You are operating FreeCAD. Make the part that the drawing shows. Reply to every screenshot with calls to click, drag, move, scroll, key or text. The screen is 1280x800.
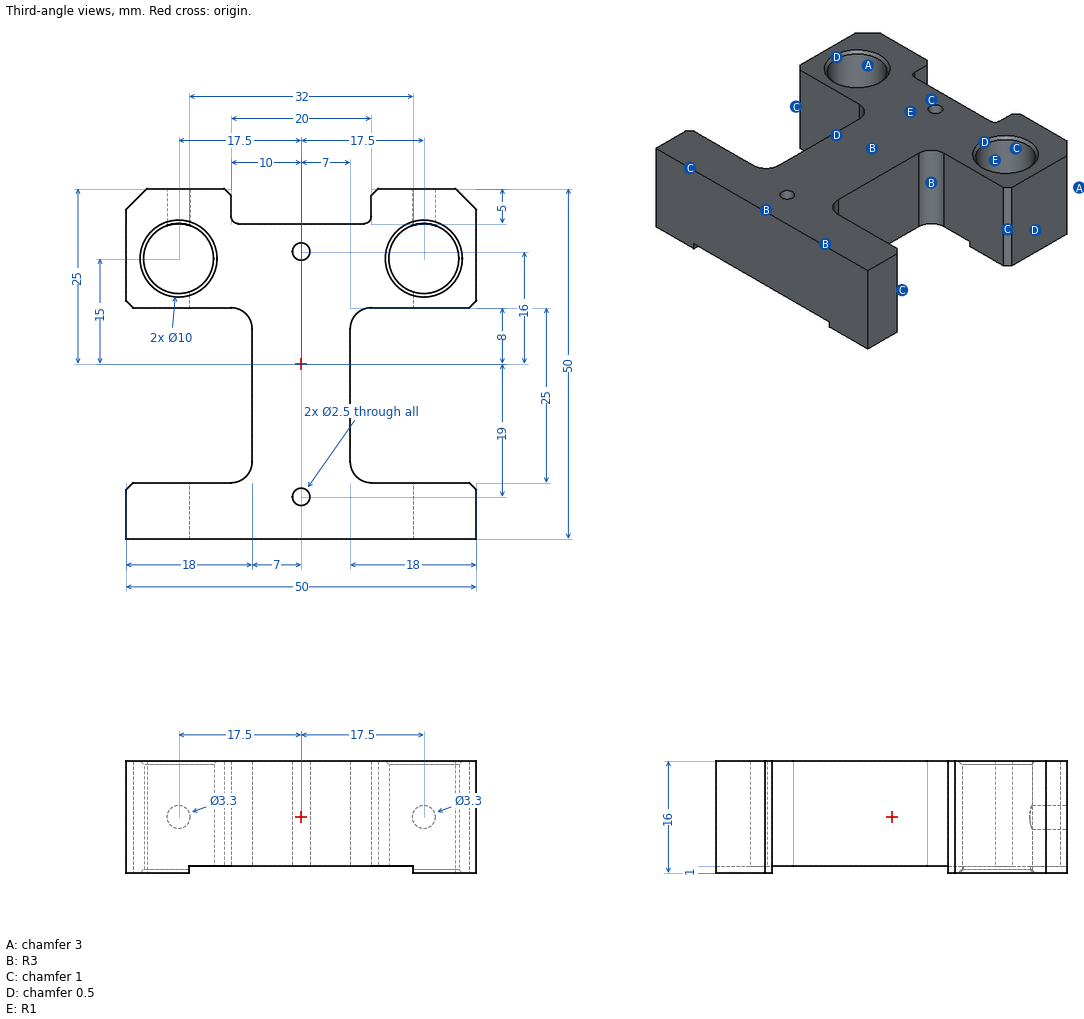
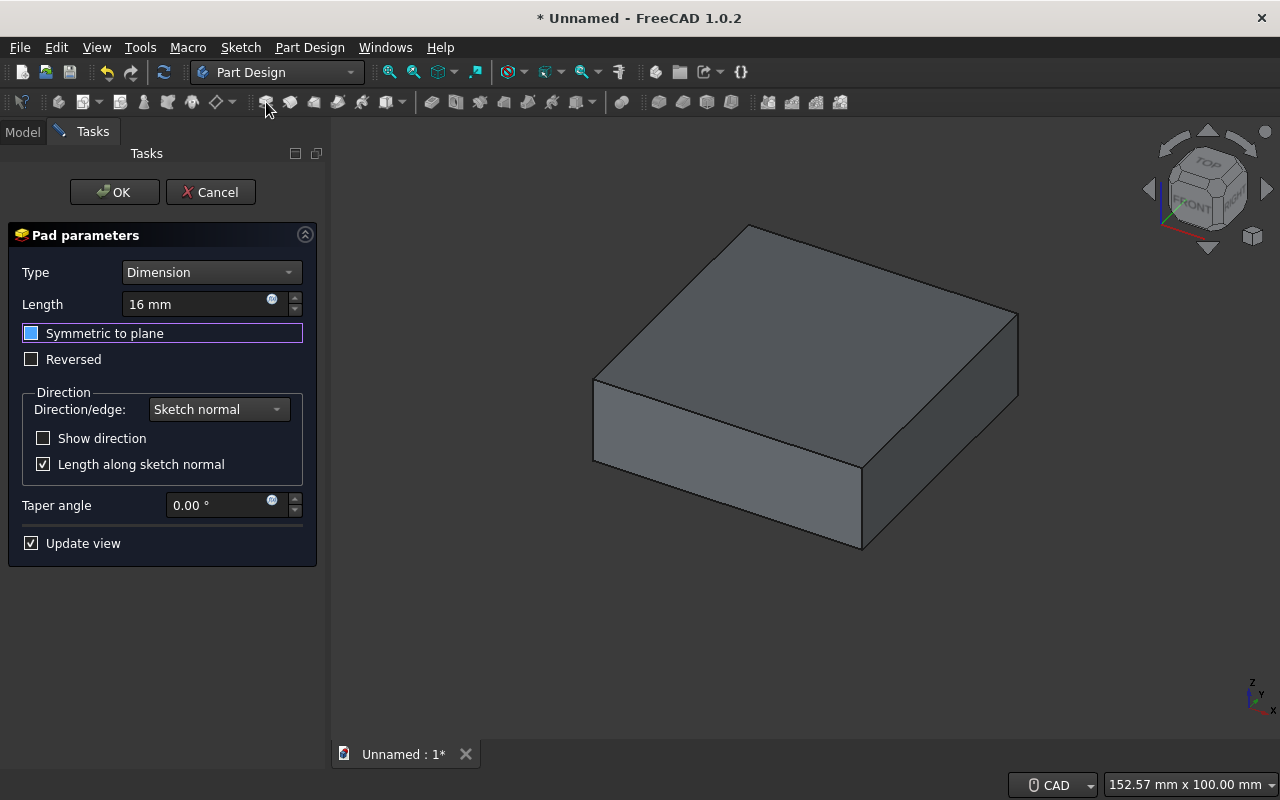
click(30, 333)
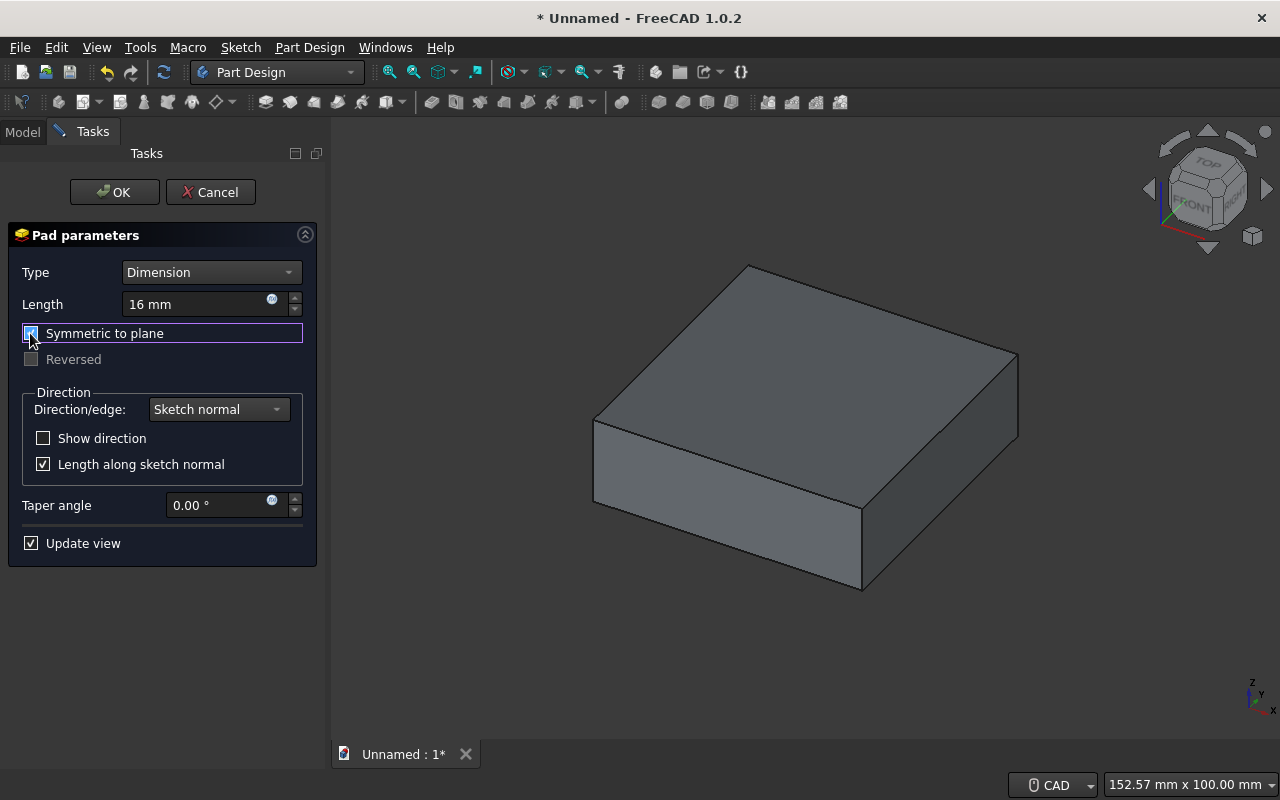
click(115, 192)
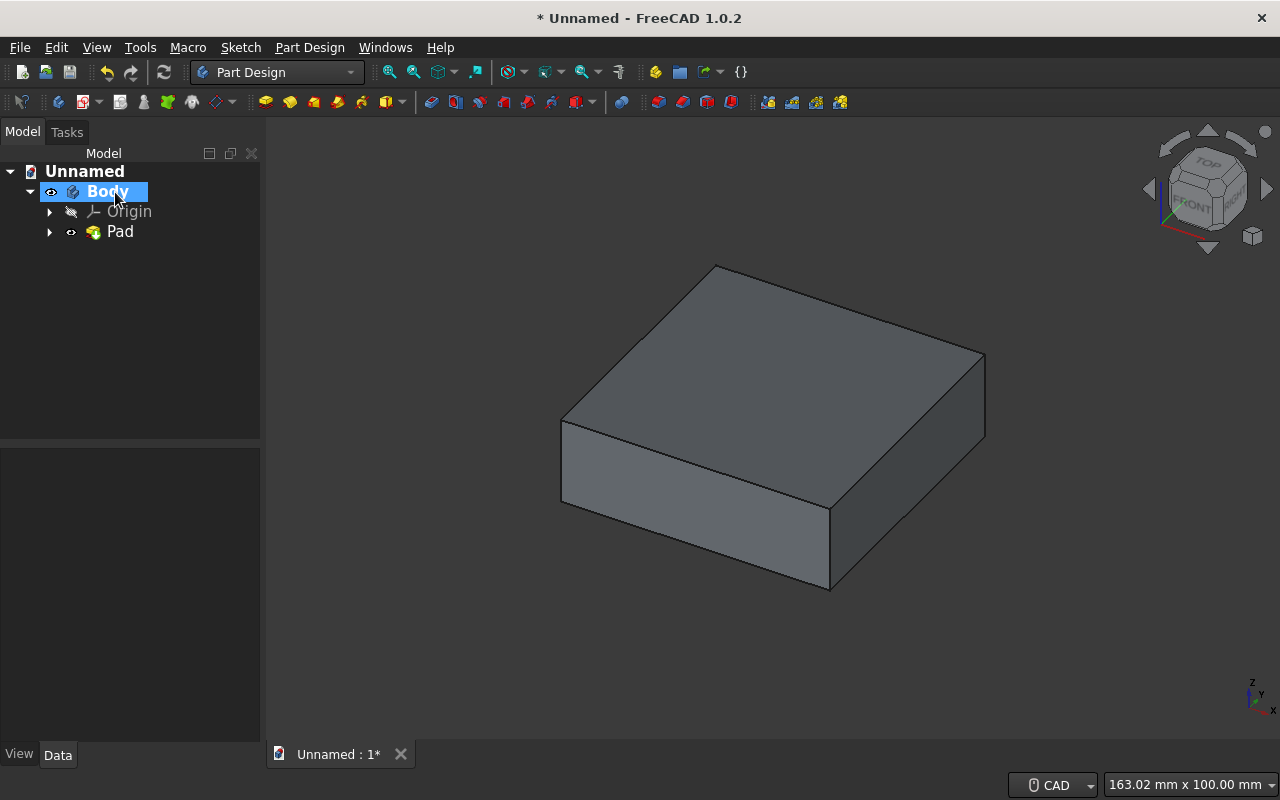
click(773, 386)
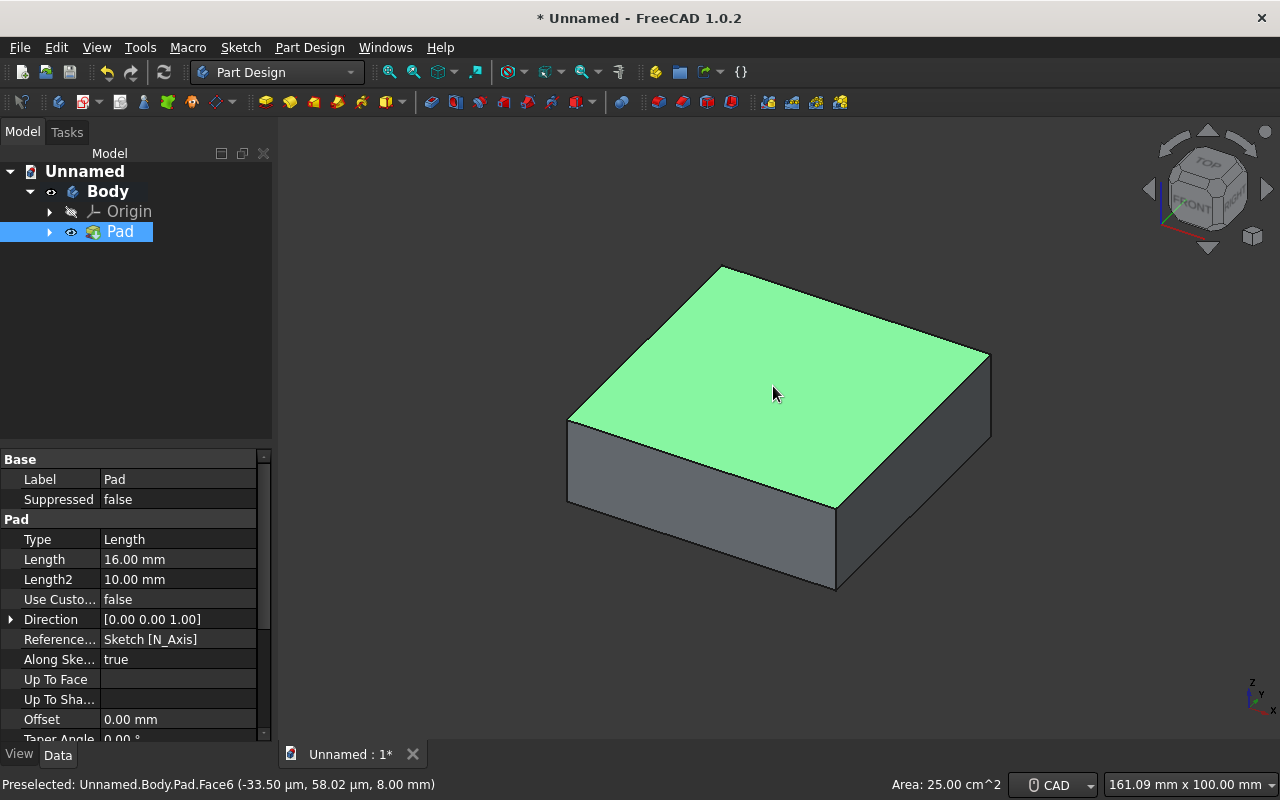
click(84, 102)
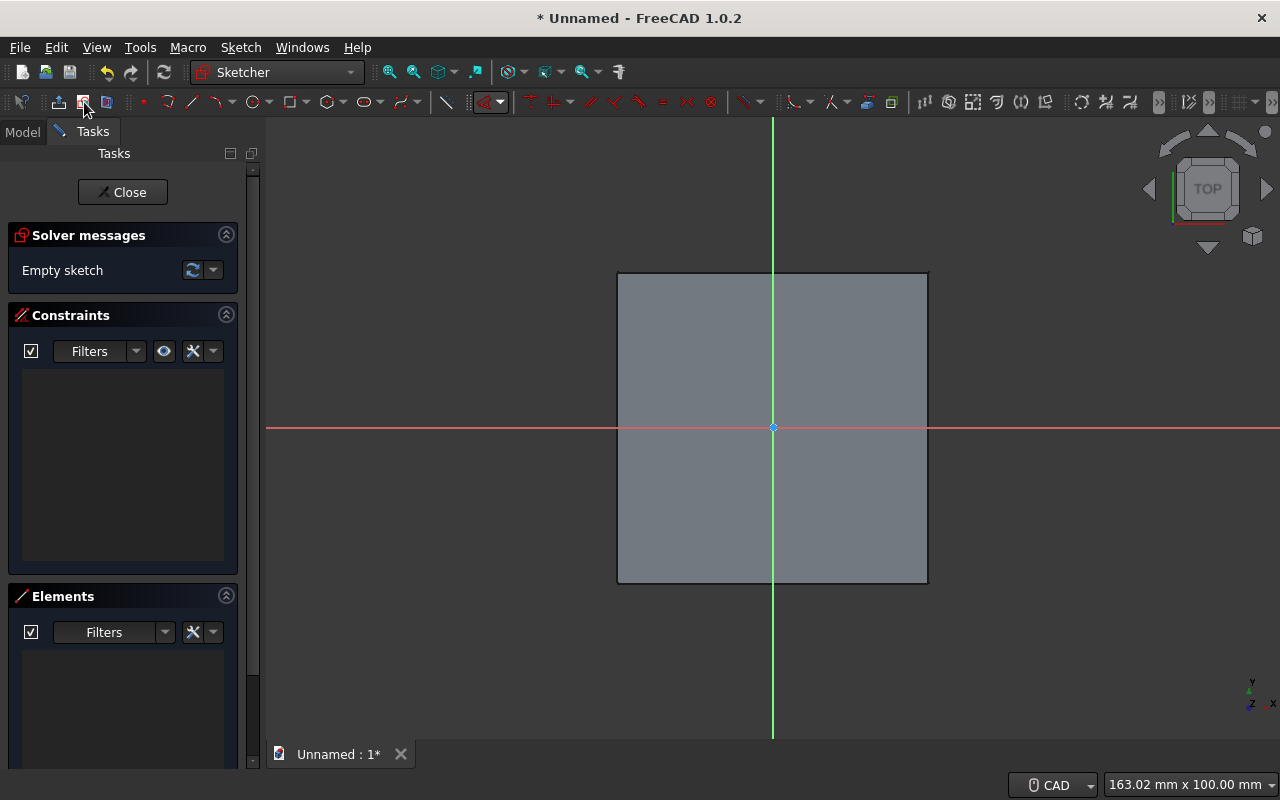
scroll(856, 407, up, 3)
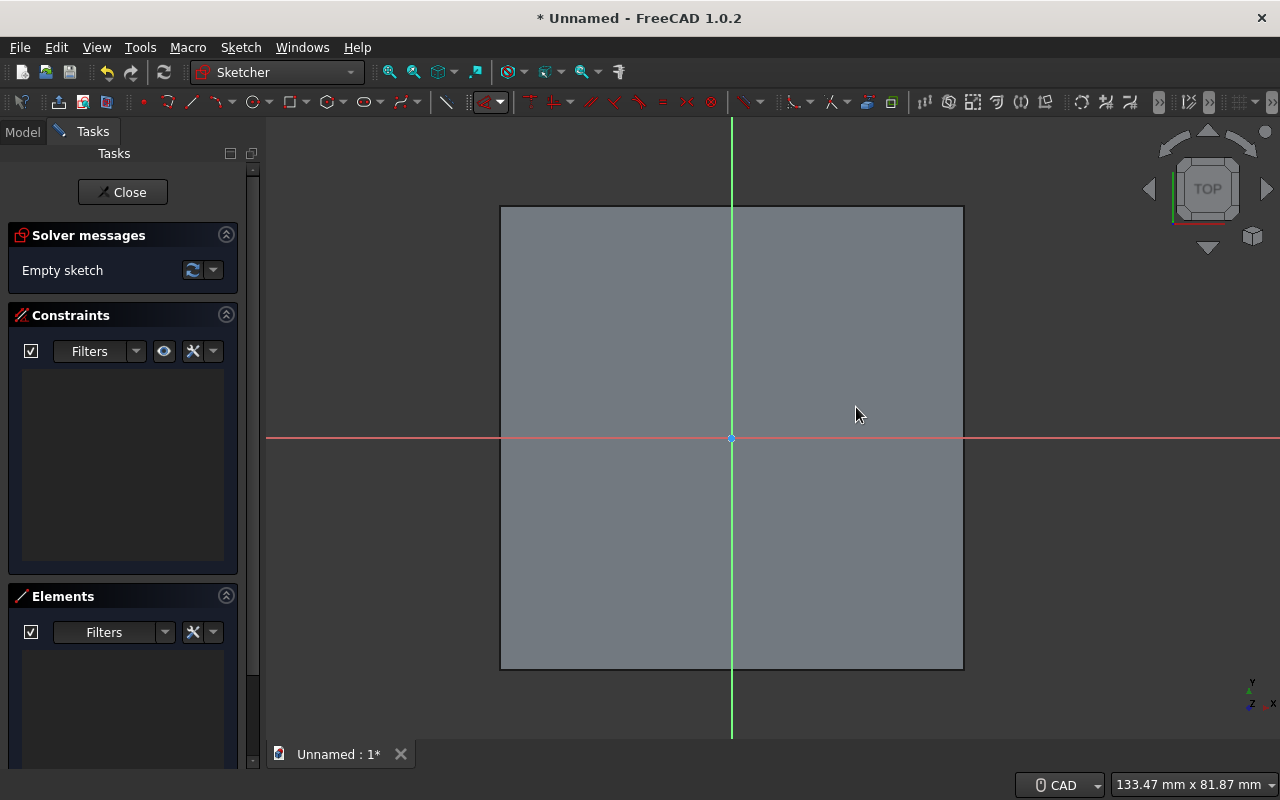
key(g)
key(r)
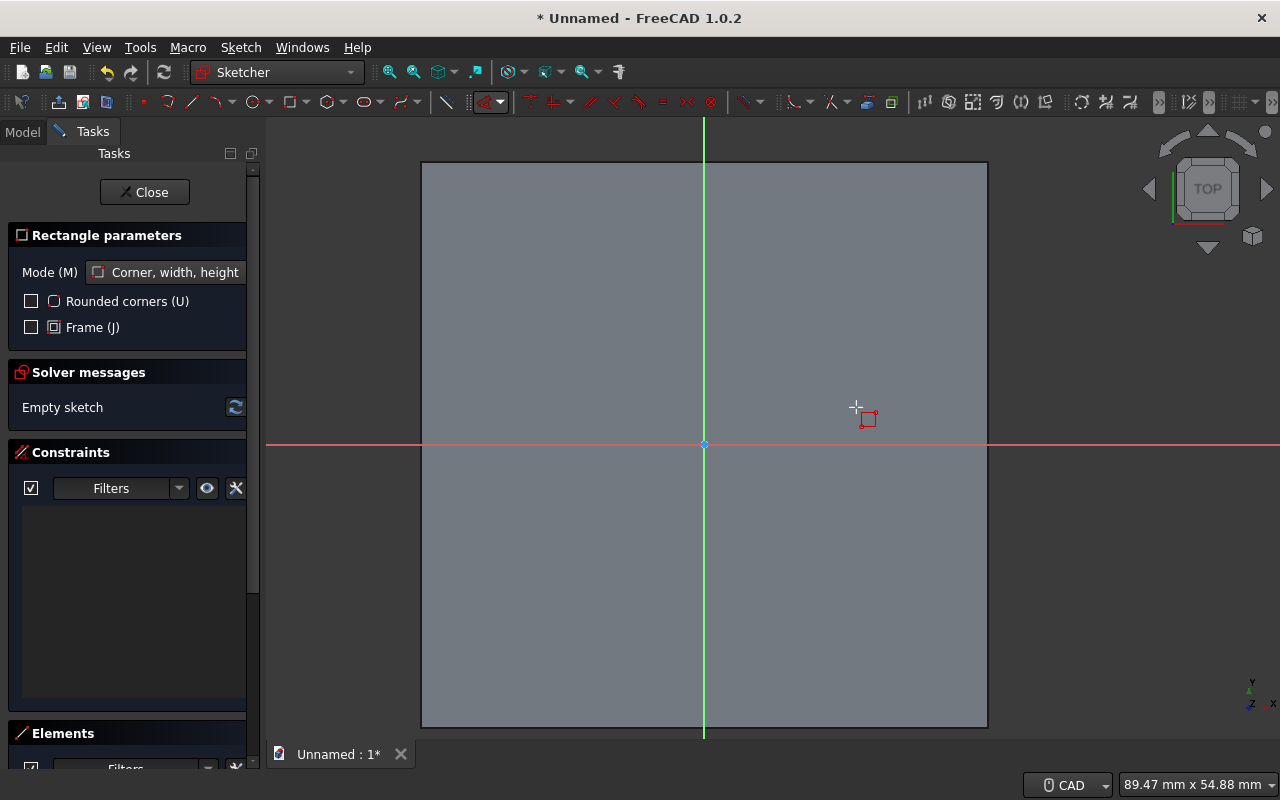
click(784, 354)
move(988, 638)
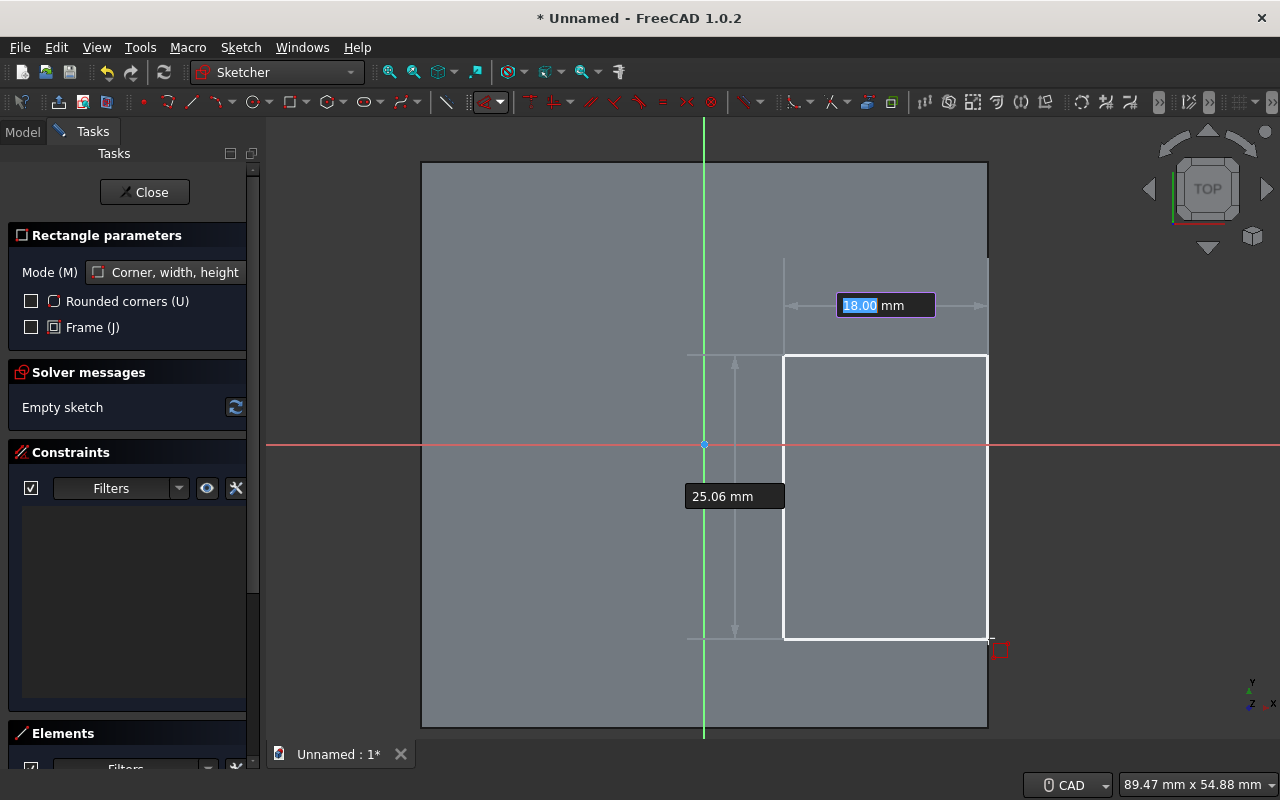
text(18)
key(Tab)
text(25)
key(Return)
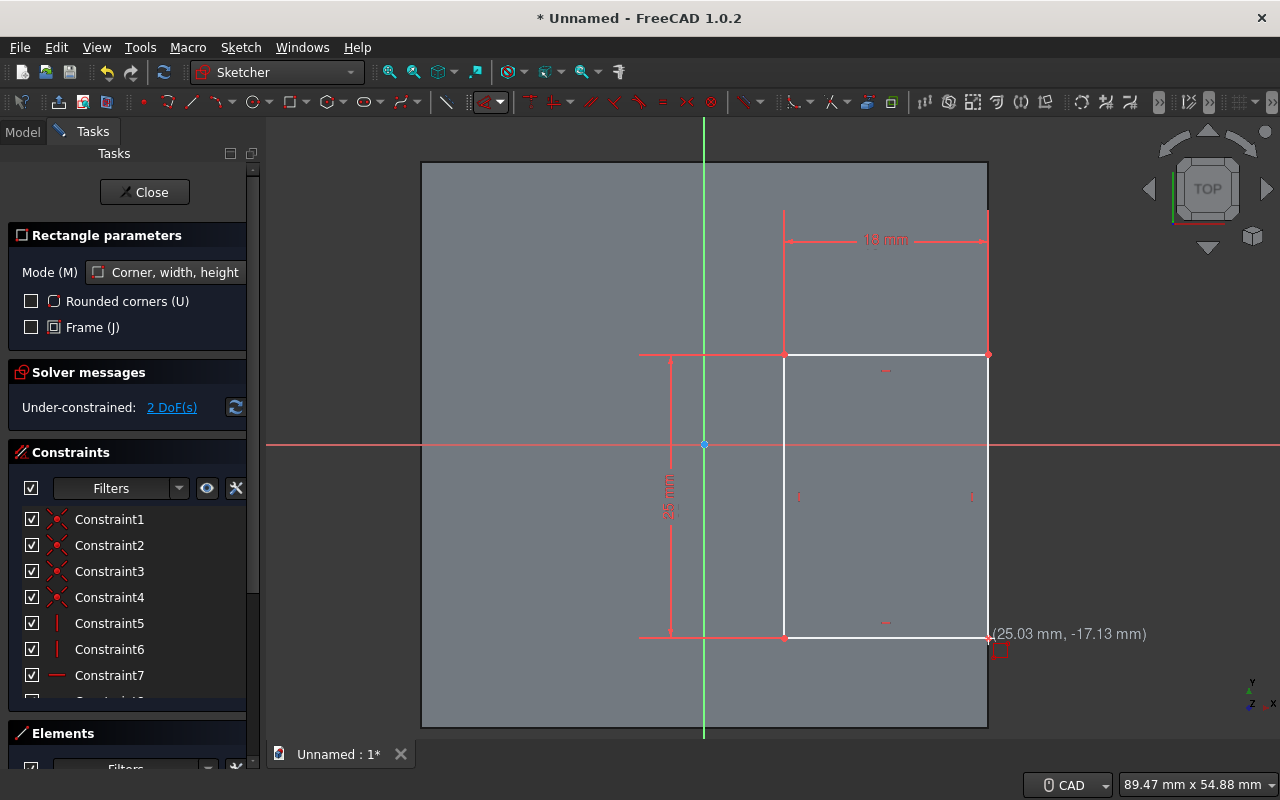
click(421, 354)
move(625, 638)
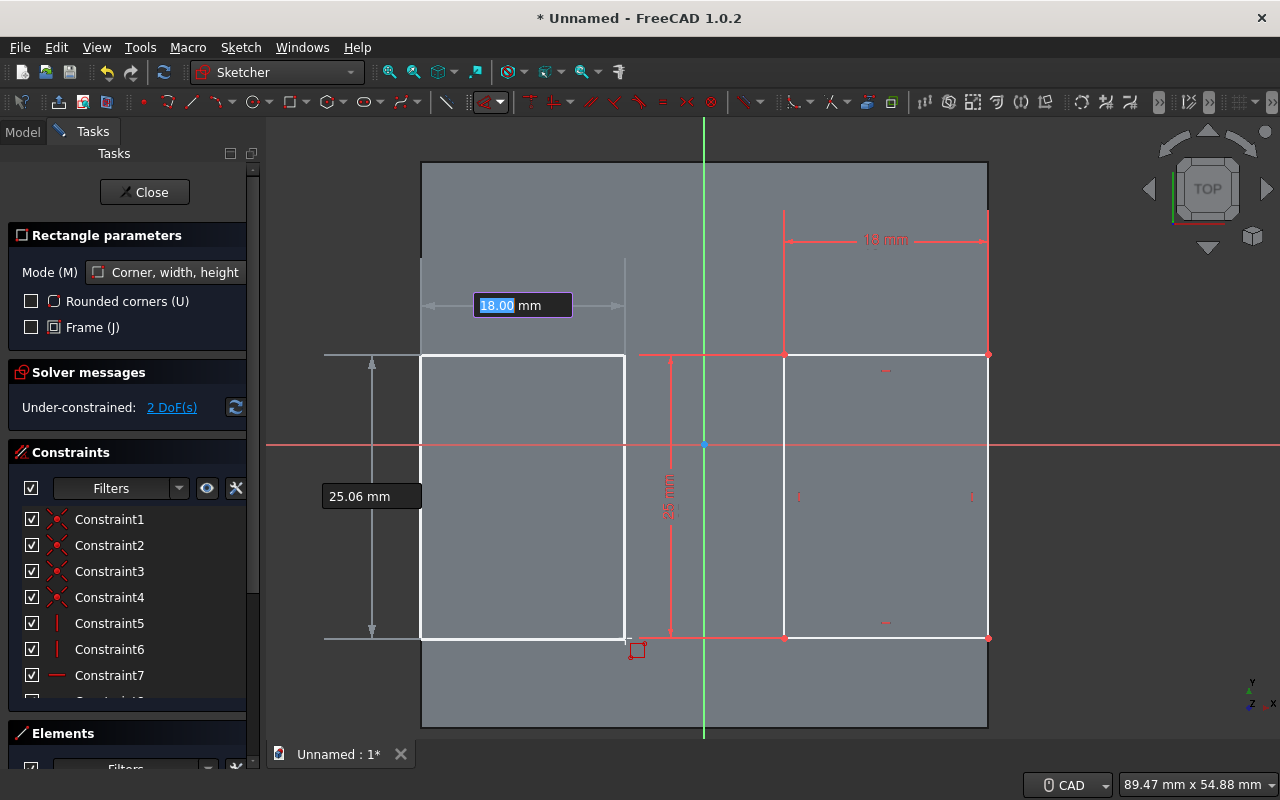
text(18)
key(Tab)
text(25)
key(Return)